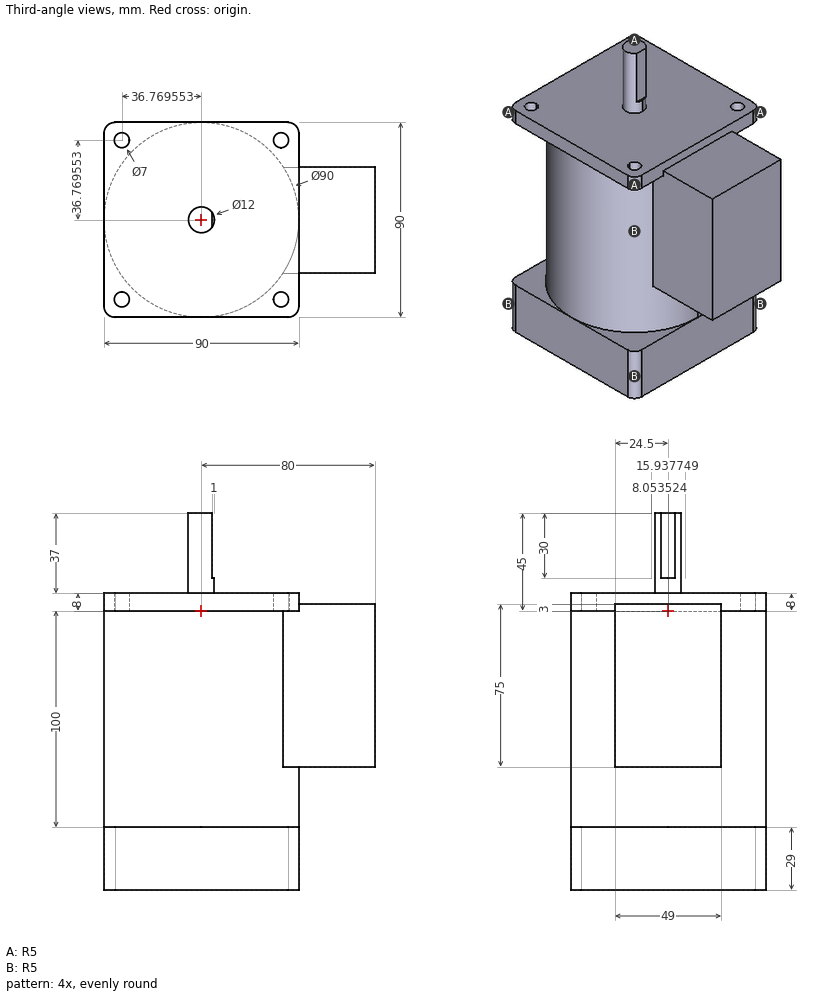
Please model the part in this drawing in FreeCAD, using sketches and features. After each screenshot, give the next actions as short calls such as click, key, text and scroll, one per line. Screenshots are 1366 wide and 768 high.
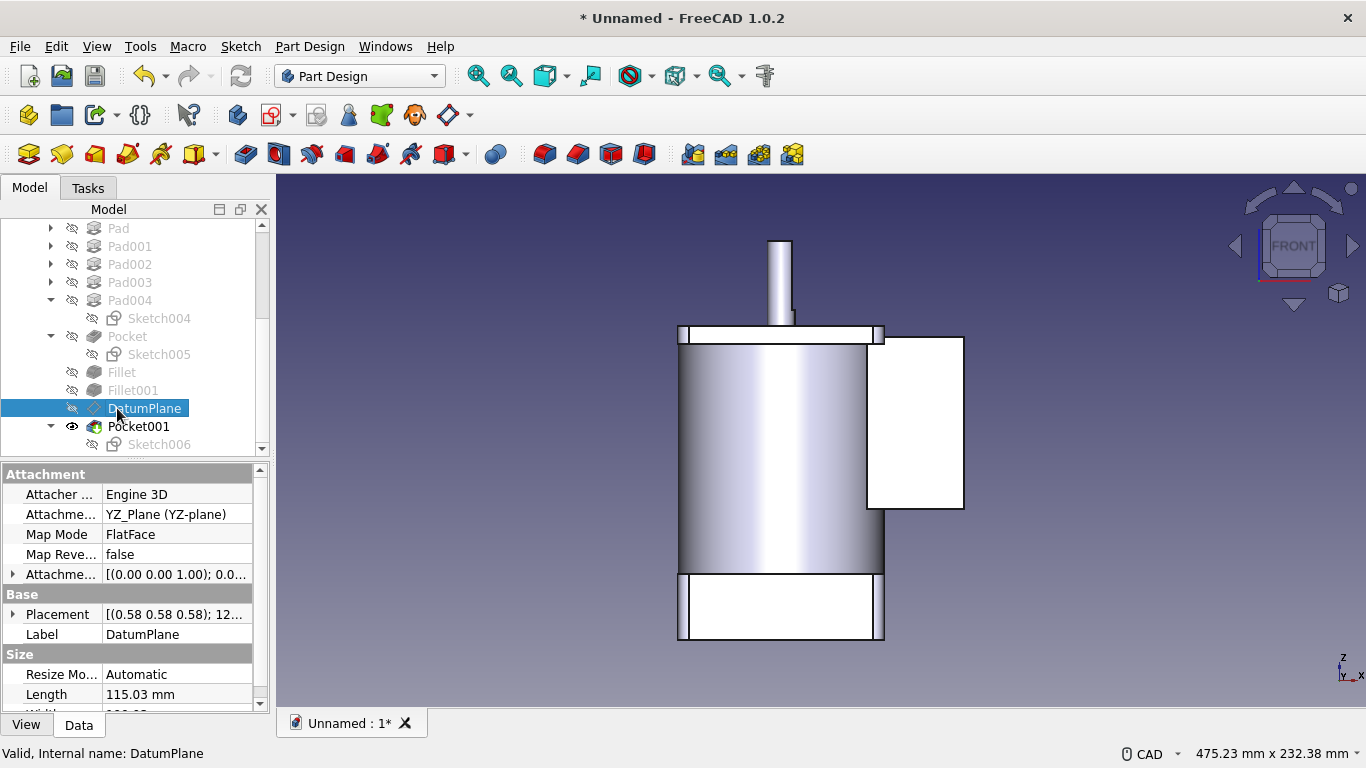
click(117, 336)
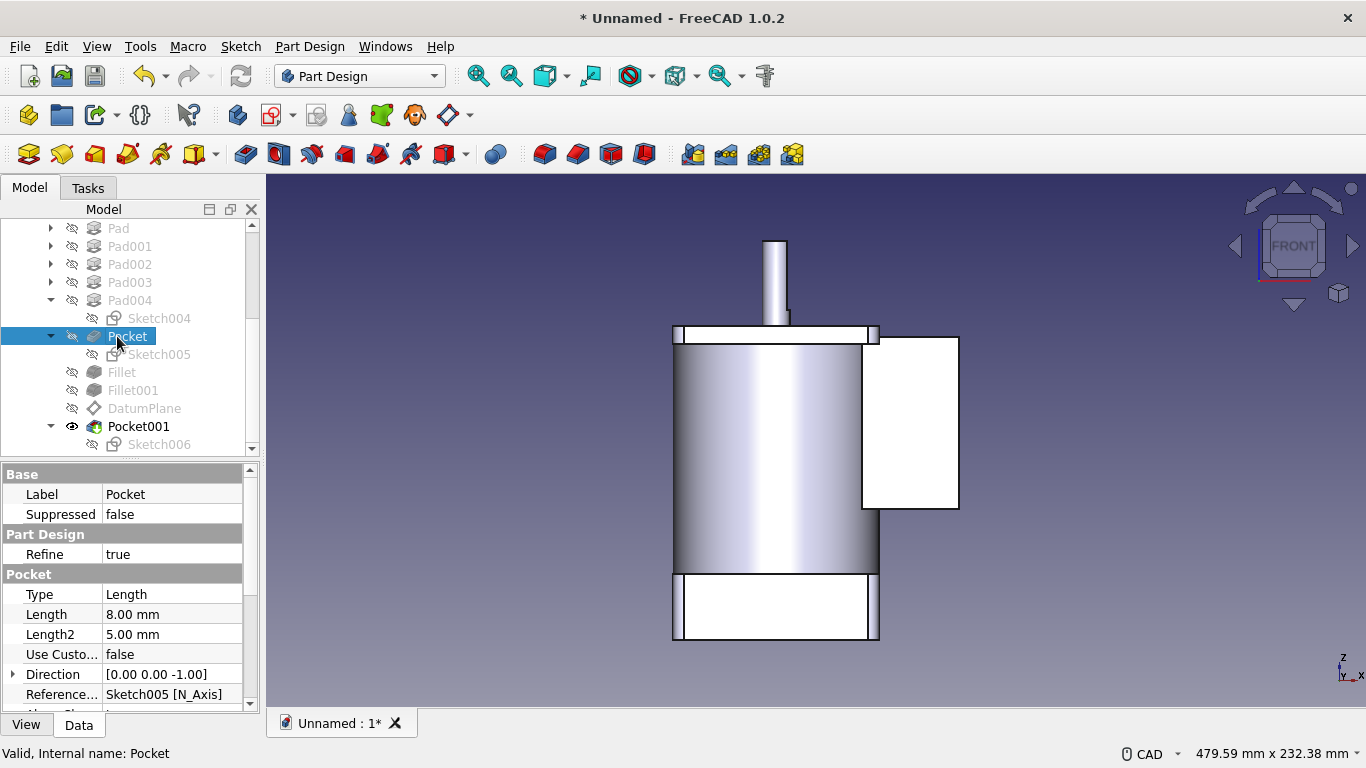
click(759, 154)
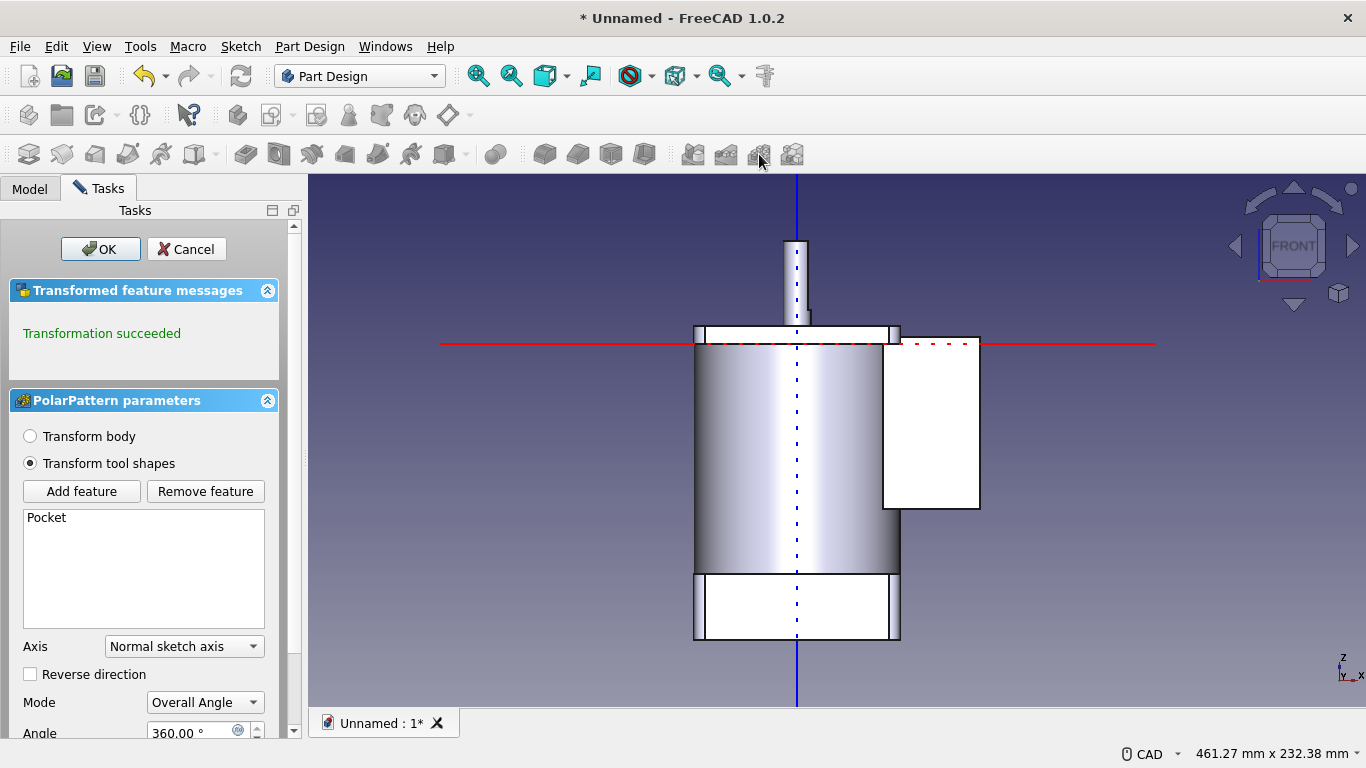
click(185, 646)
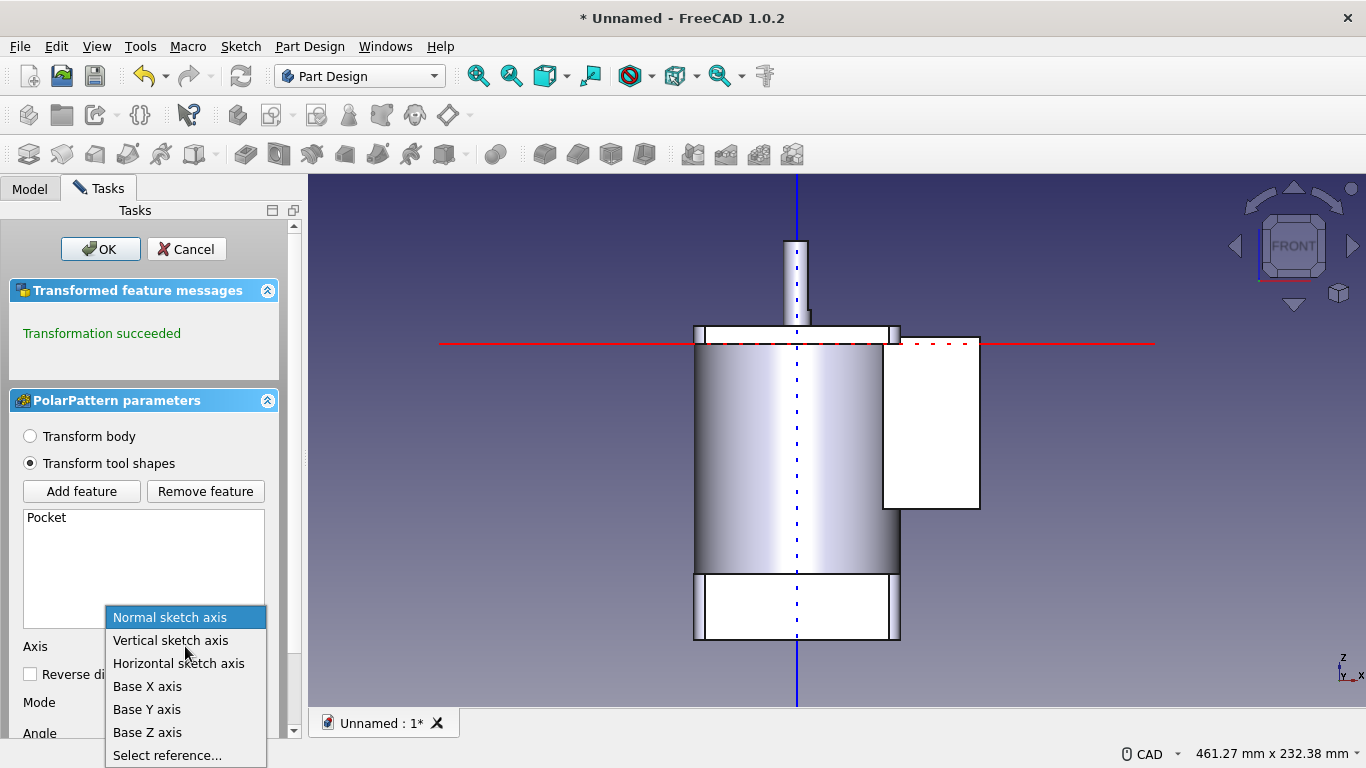
click(184, 732)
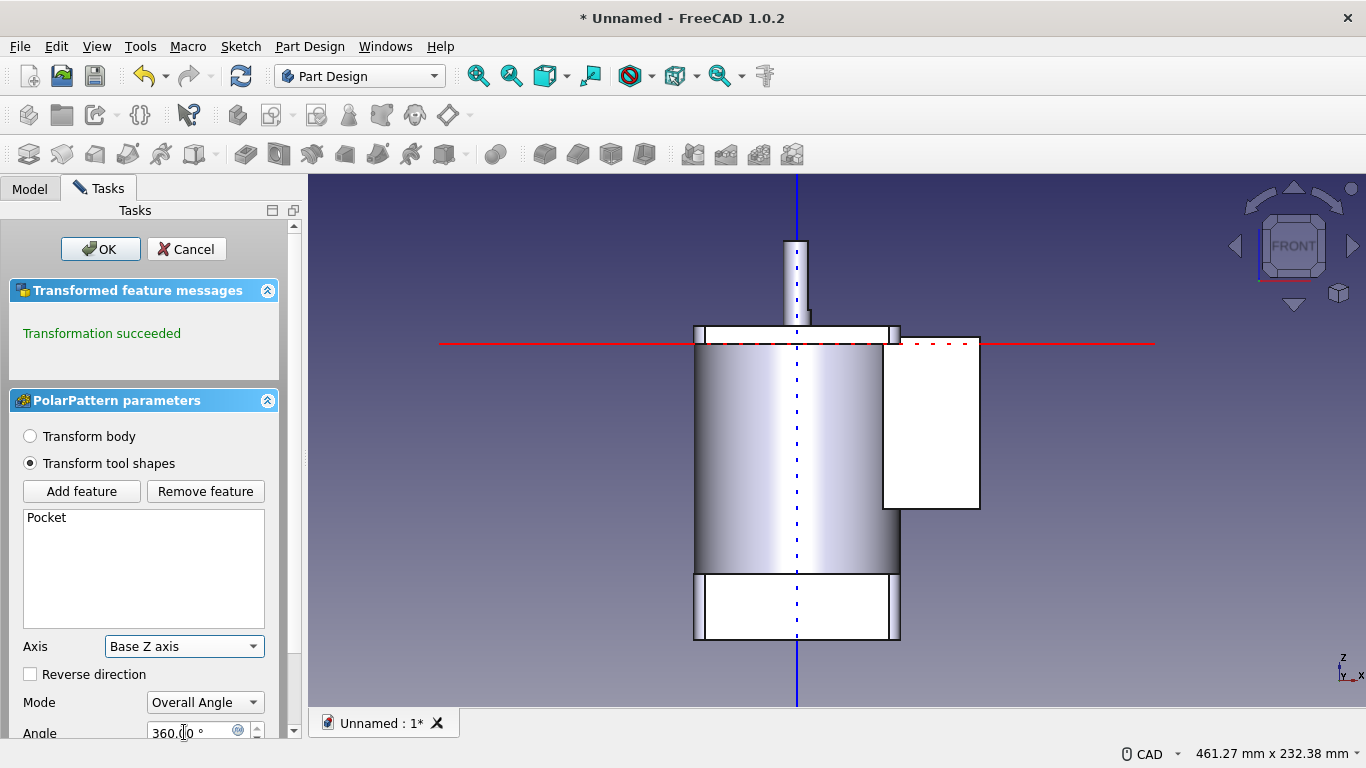
scroll(294, 479, down, 2)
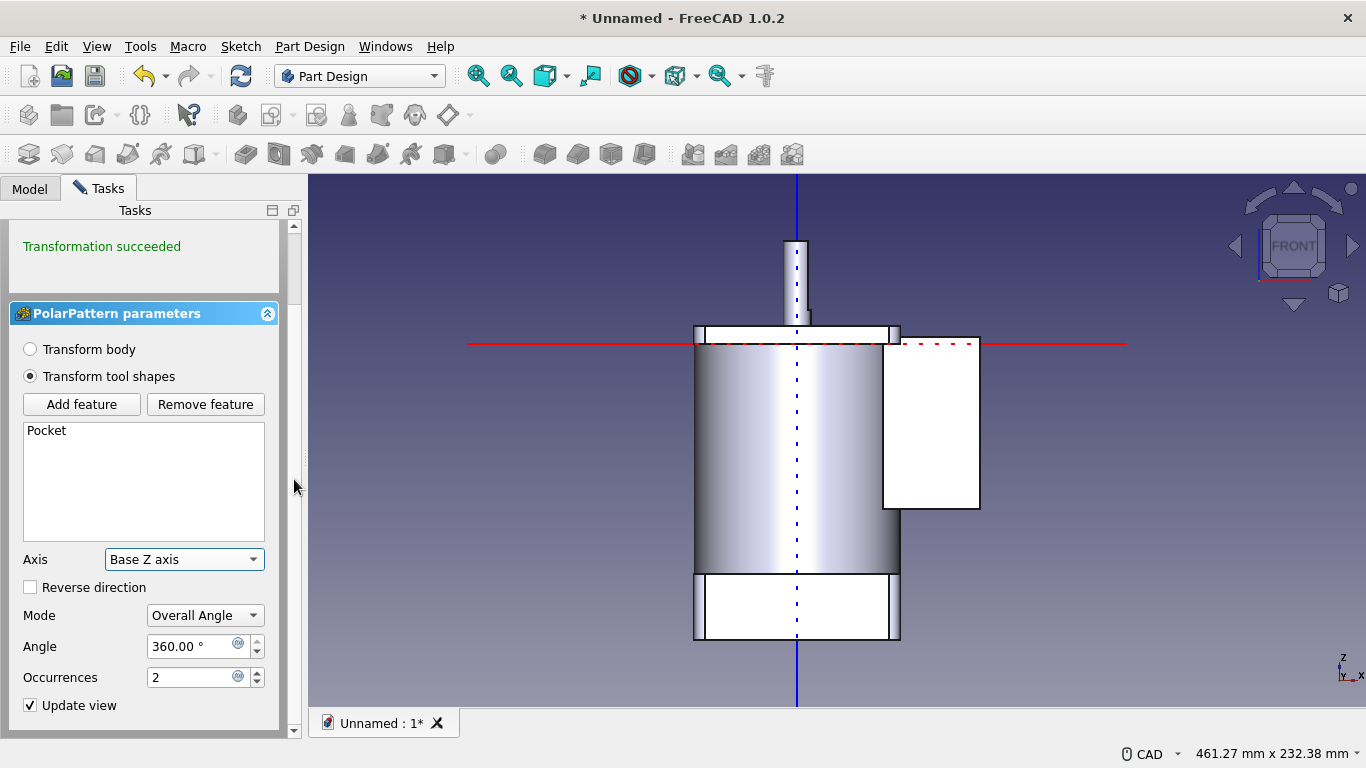
triple_click(199, 678)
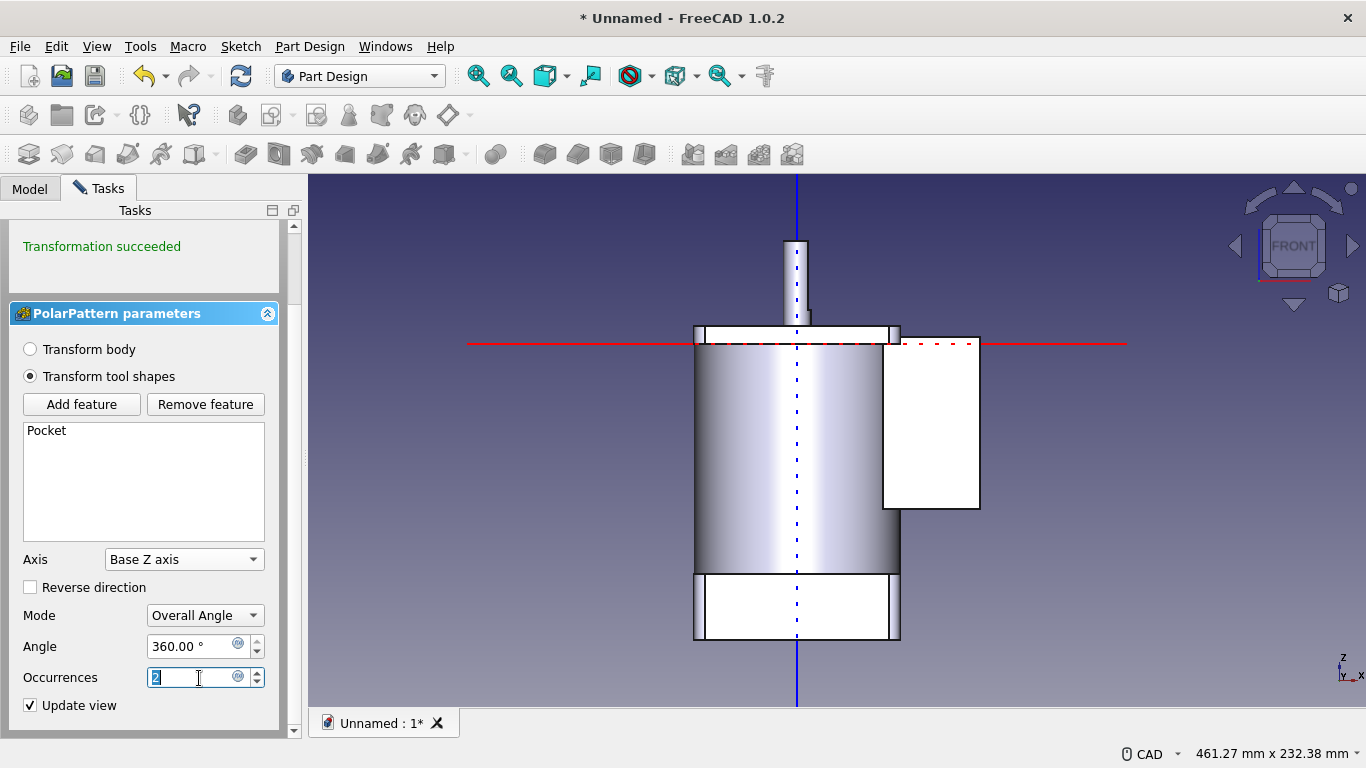
text(4)
key(Tab)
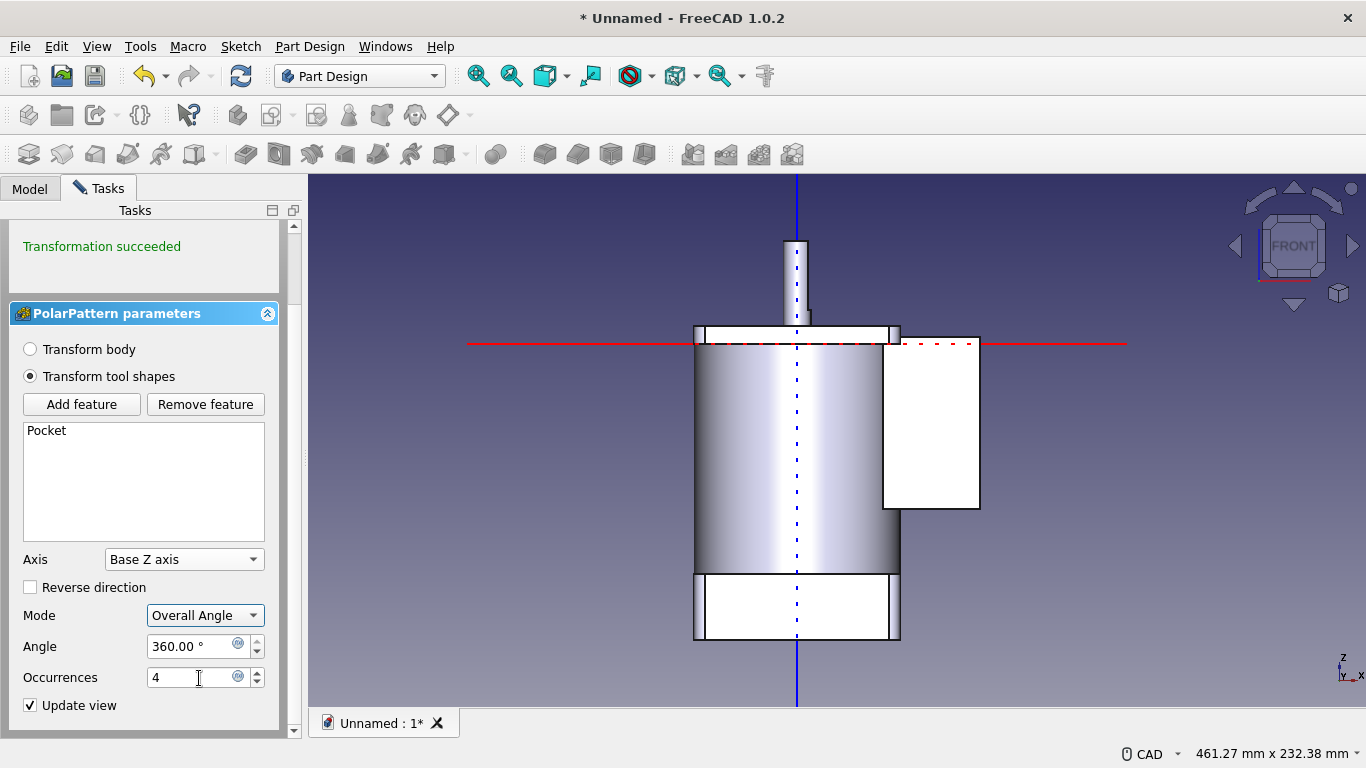
scroll(294, 479, up, 3)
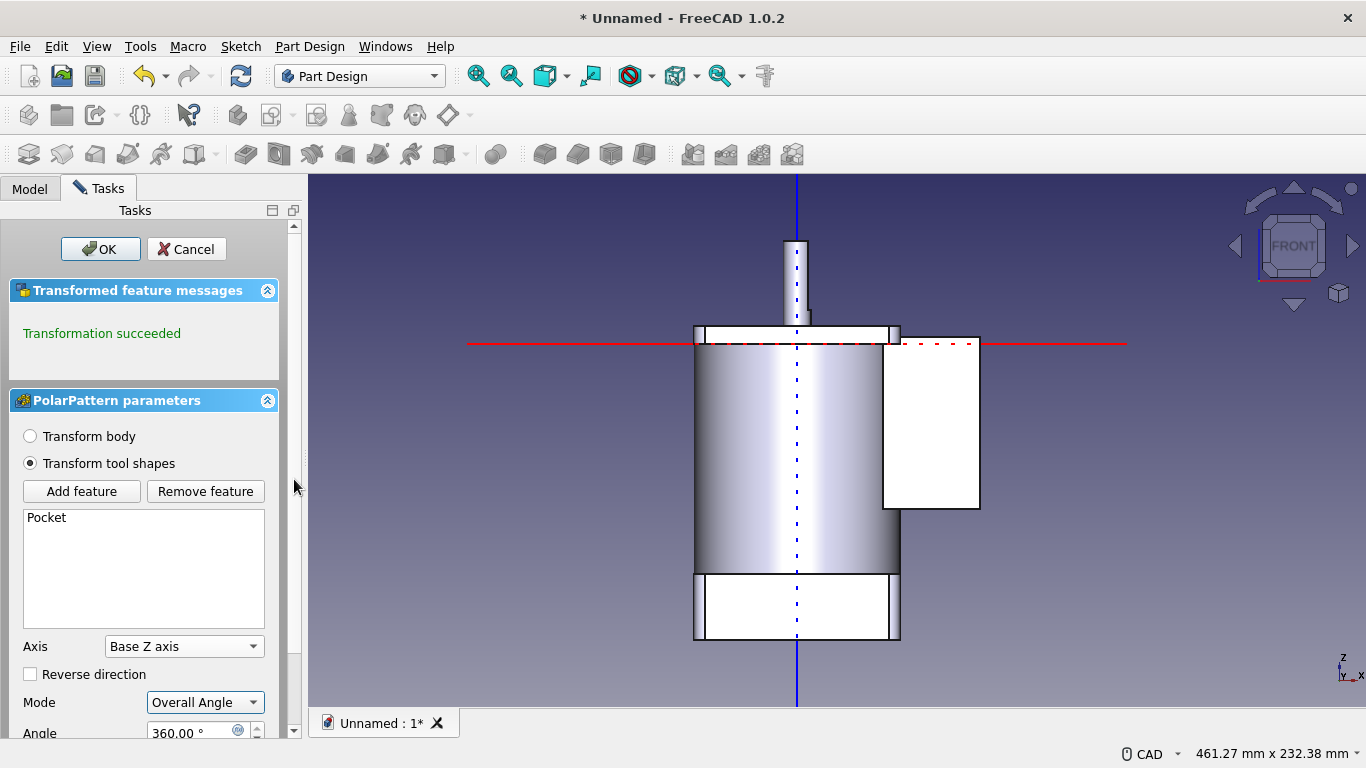
click(101, 249)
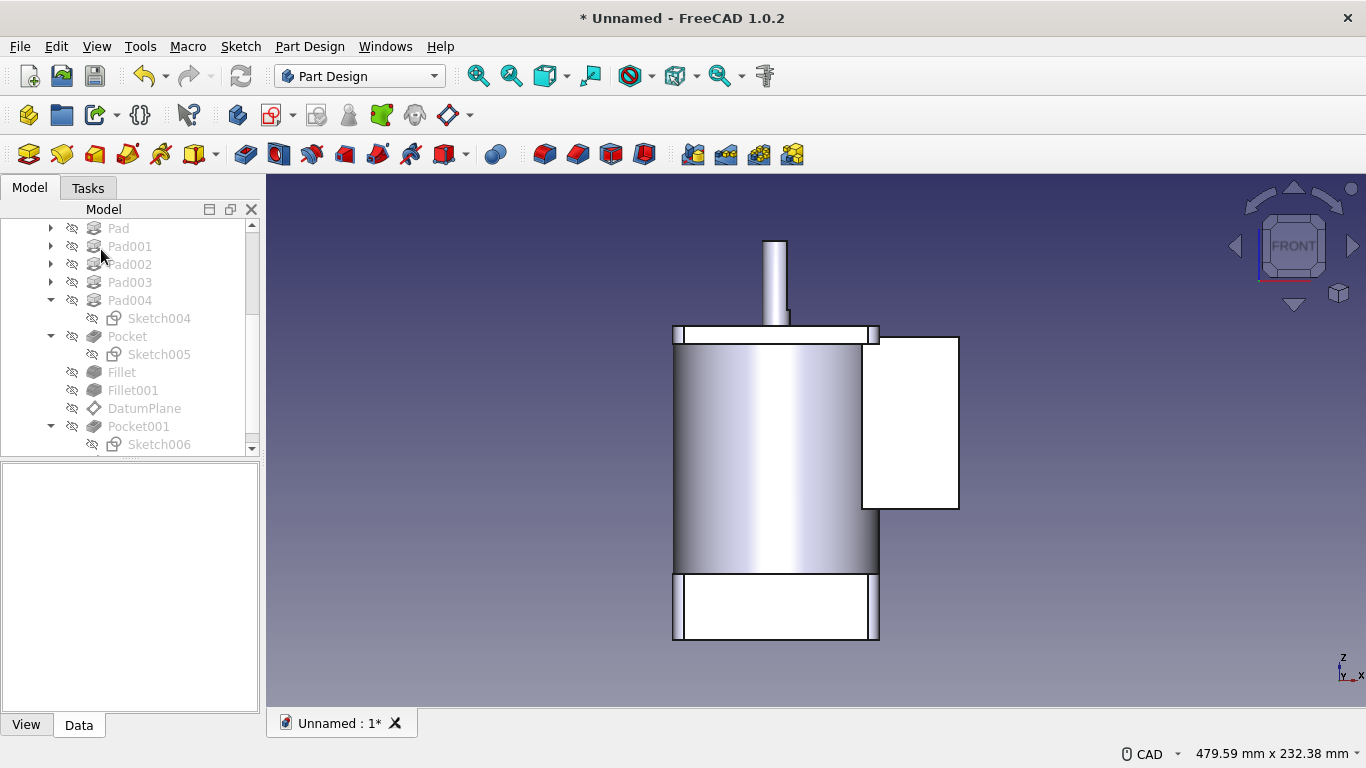
key(0)